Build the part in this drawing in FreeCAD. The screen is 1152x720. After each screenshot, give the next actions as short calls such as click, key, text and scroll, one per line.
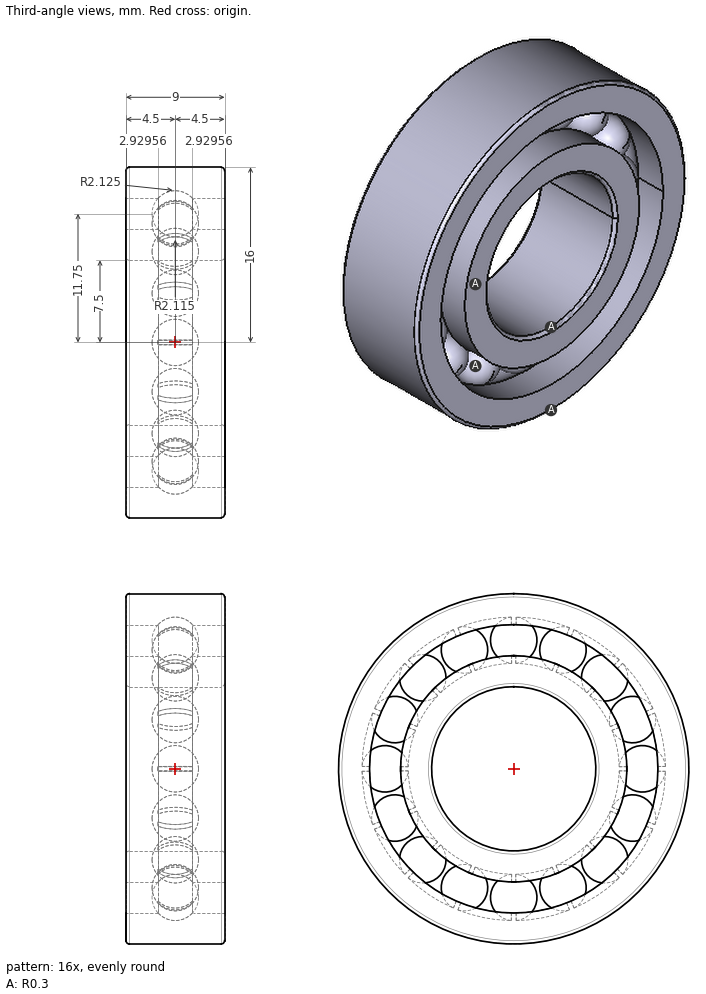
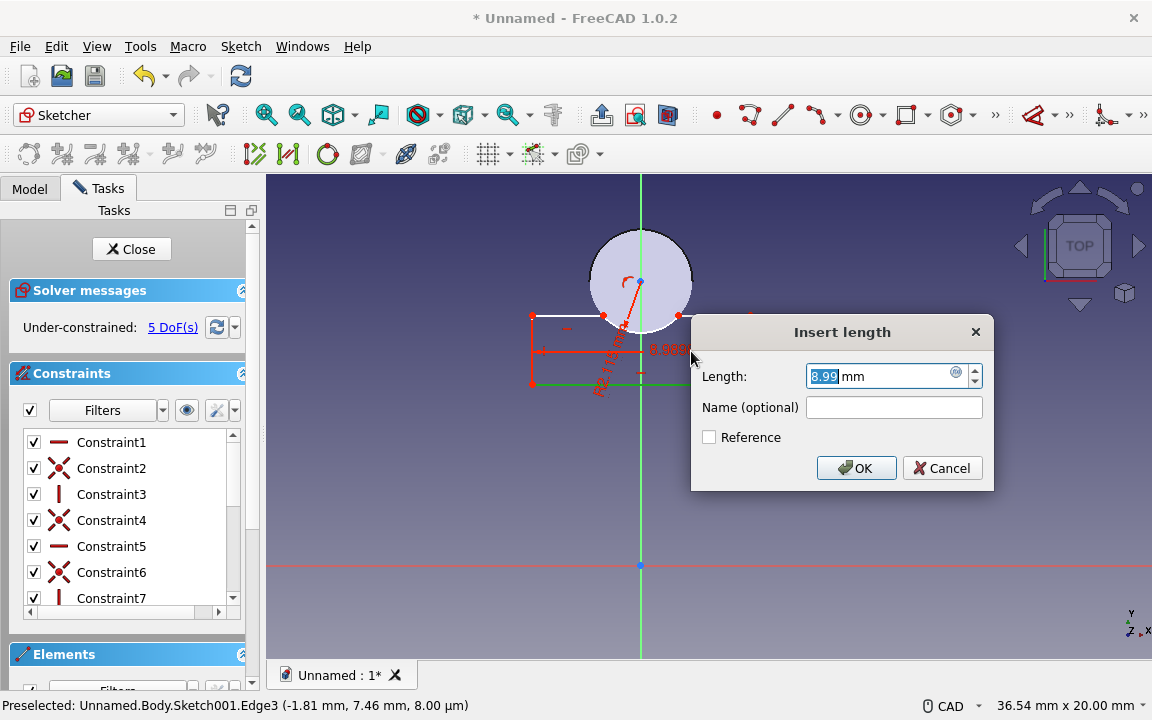
text(9)
key(Return)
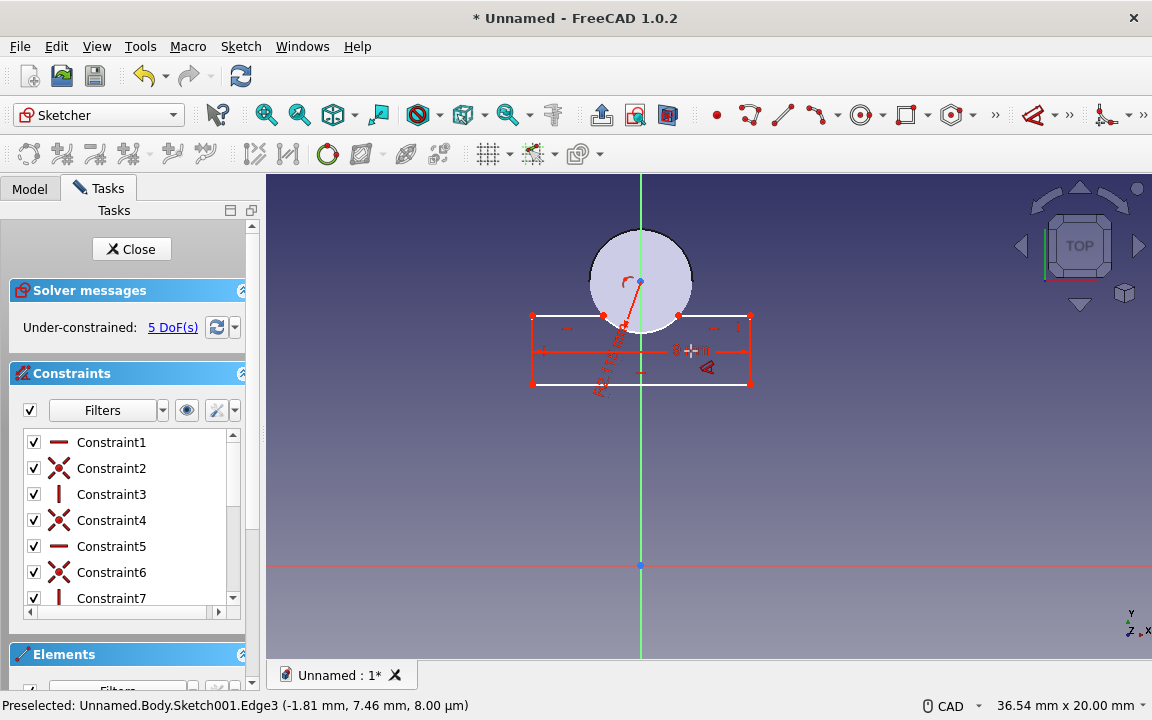
click(532, 316)
click(586, 600)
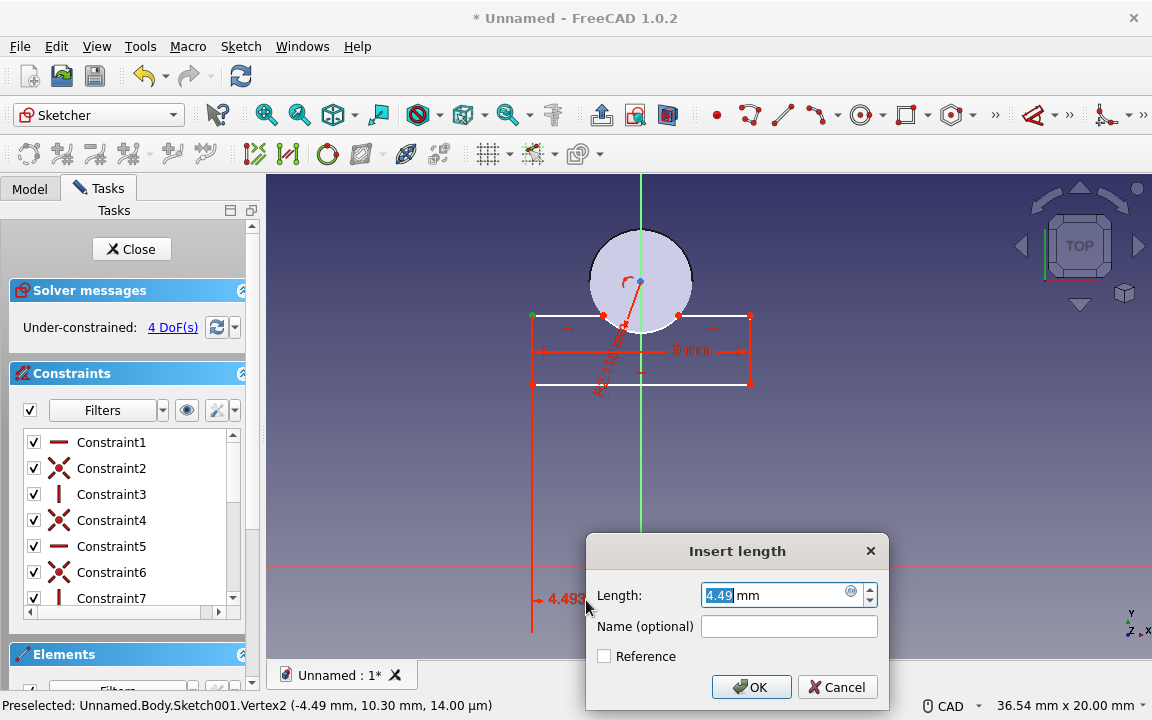
text(4.5)
key(Return)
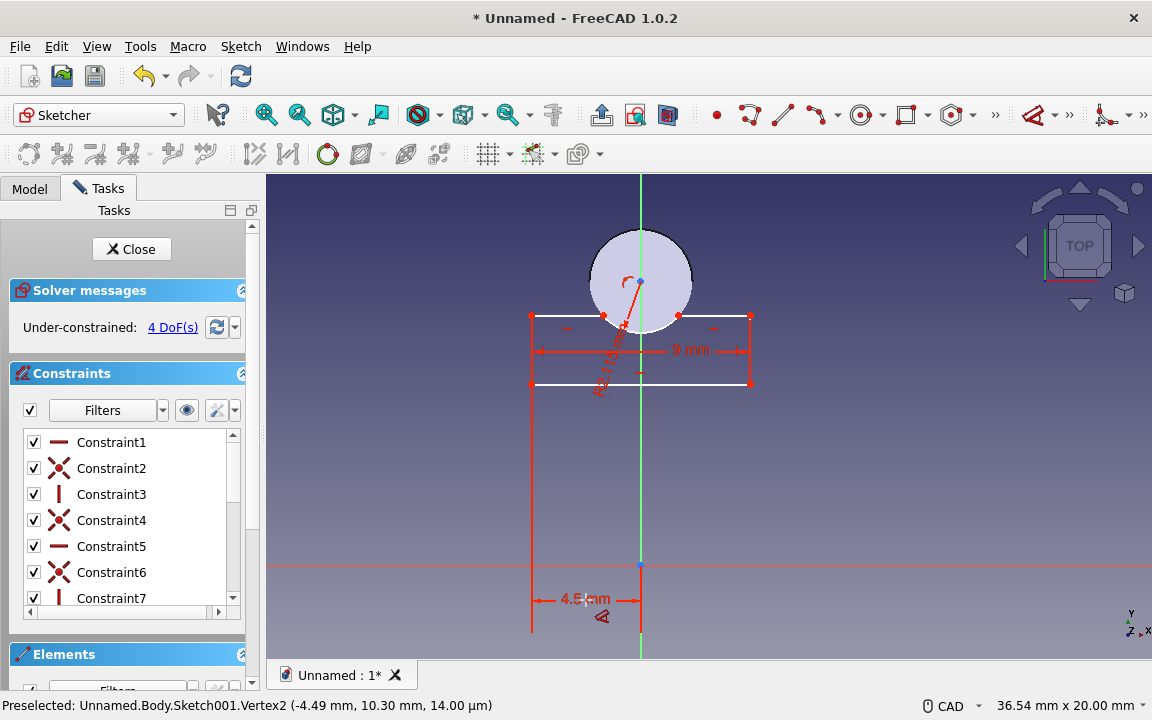
click(532, 385)
click(498, 475)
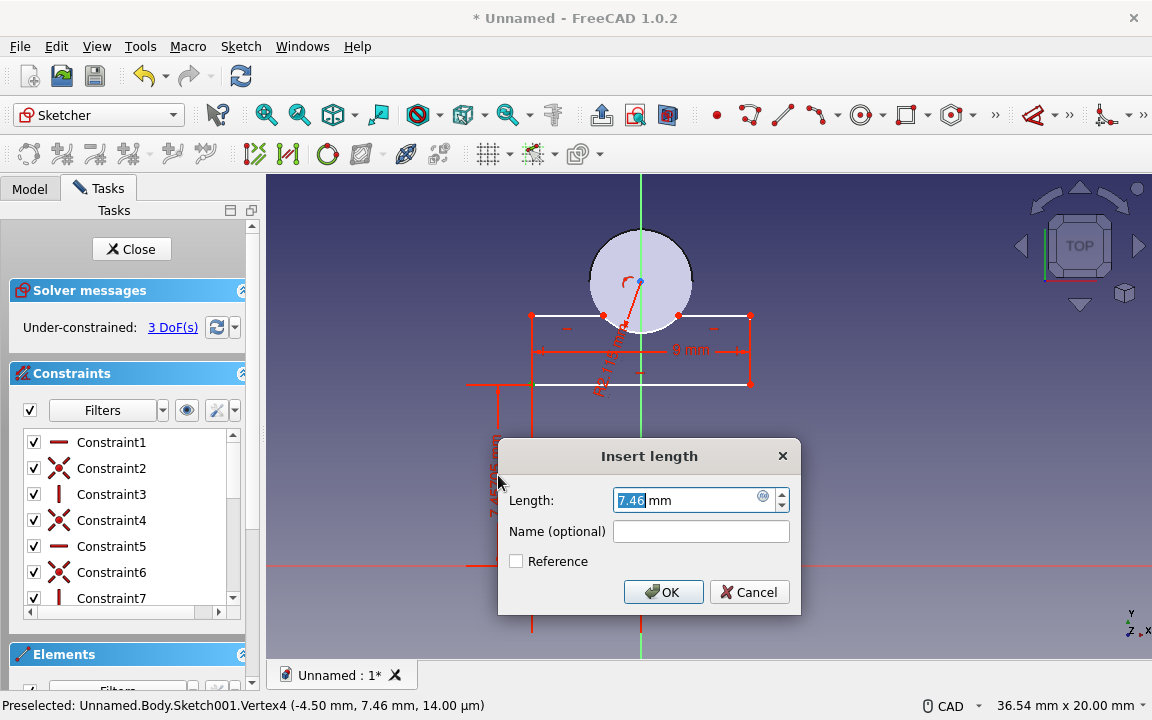
text(7.5)
key(Return)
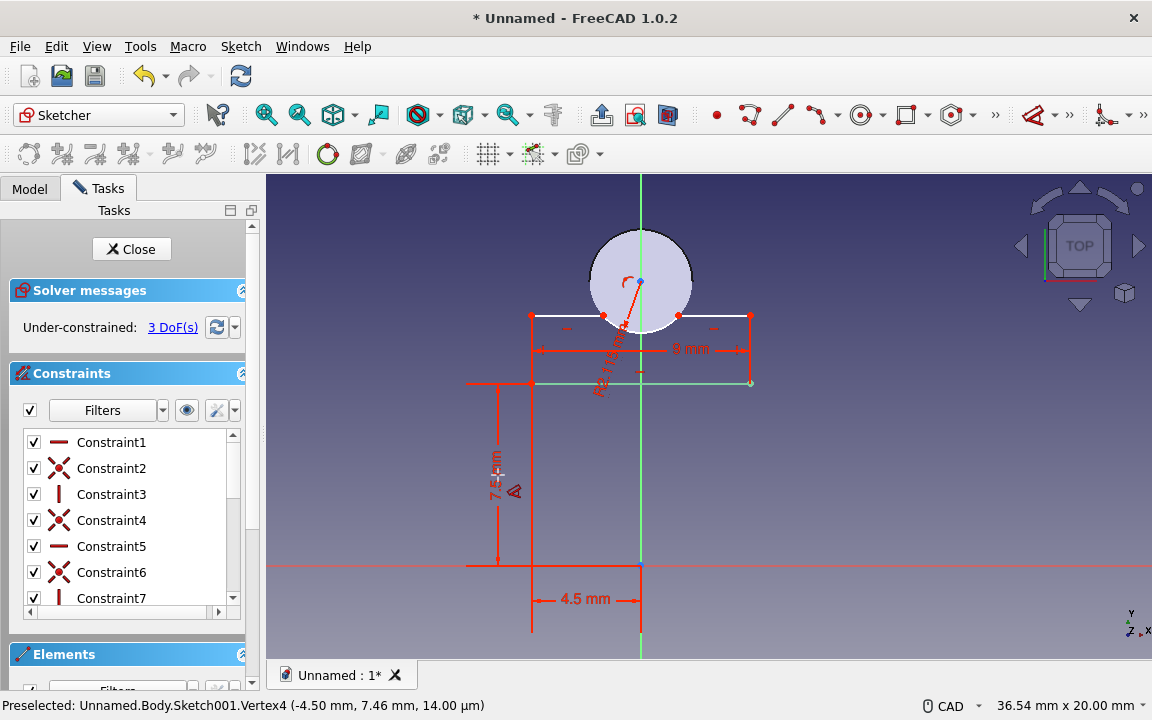
click(641, 282)
click(675, 424)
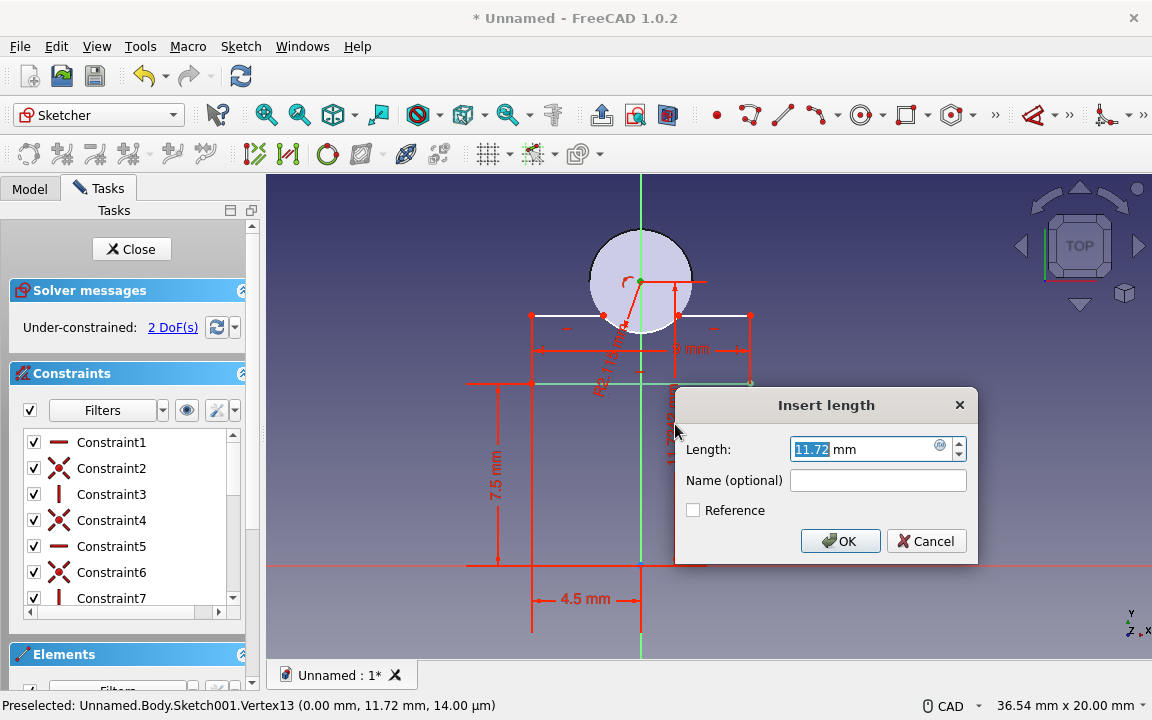
text(11.75)
key(Return)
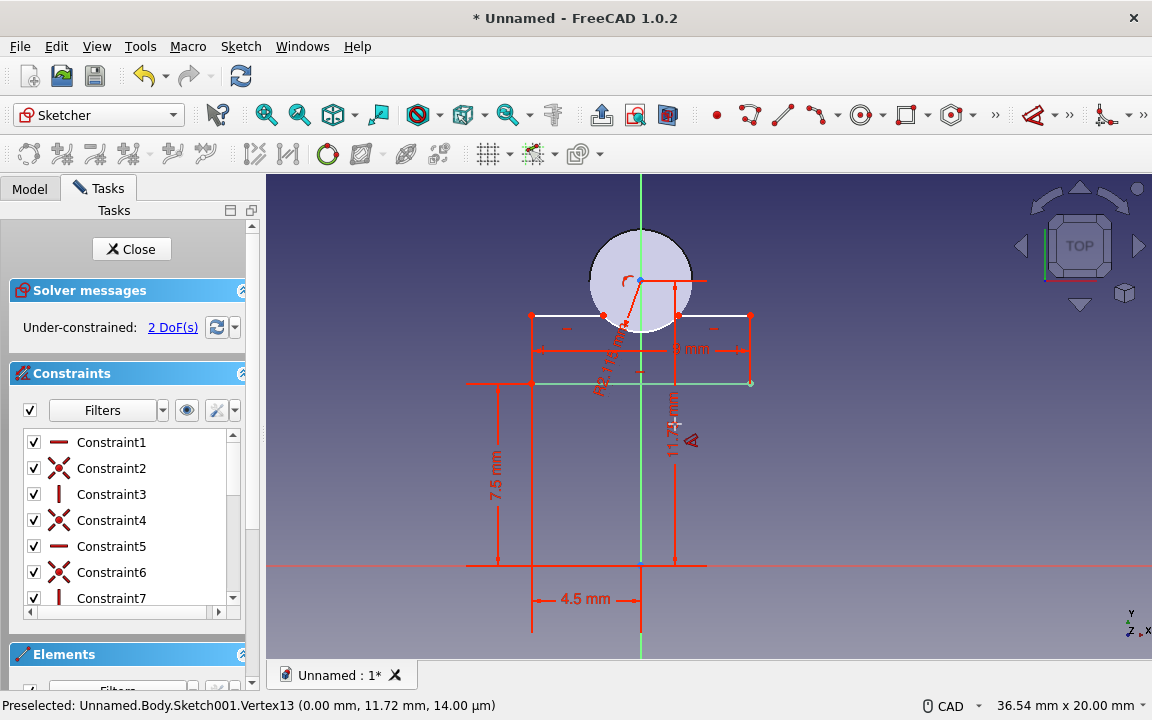
click(582, 316)
click(568, 282)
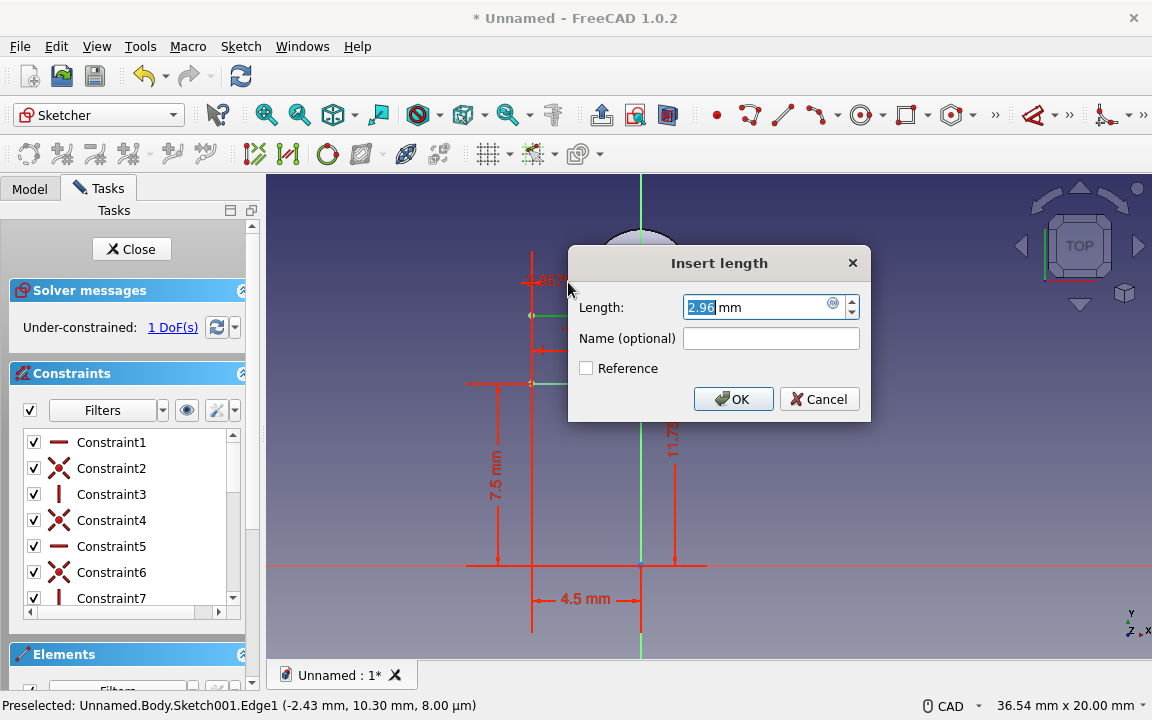
text(2.92956)
key(Return)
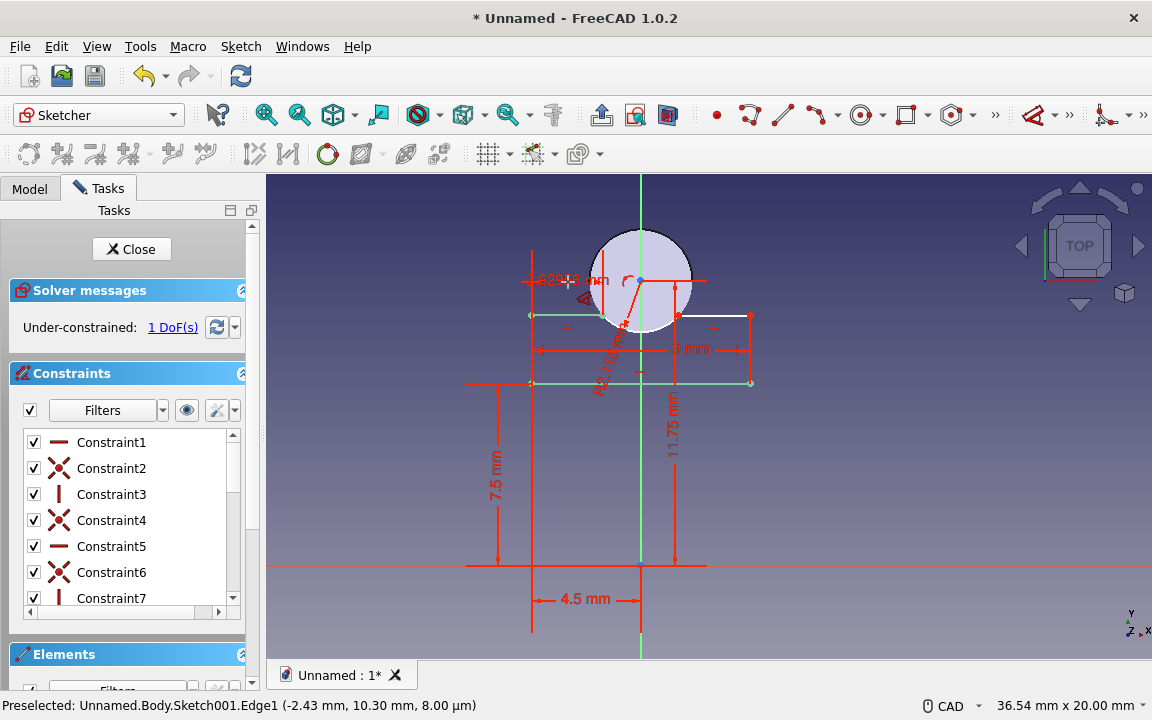
click(729, 316)
click(714, 282)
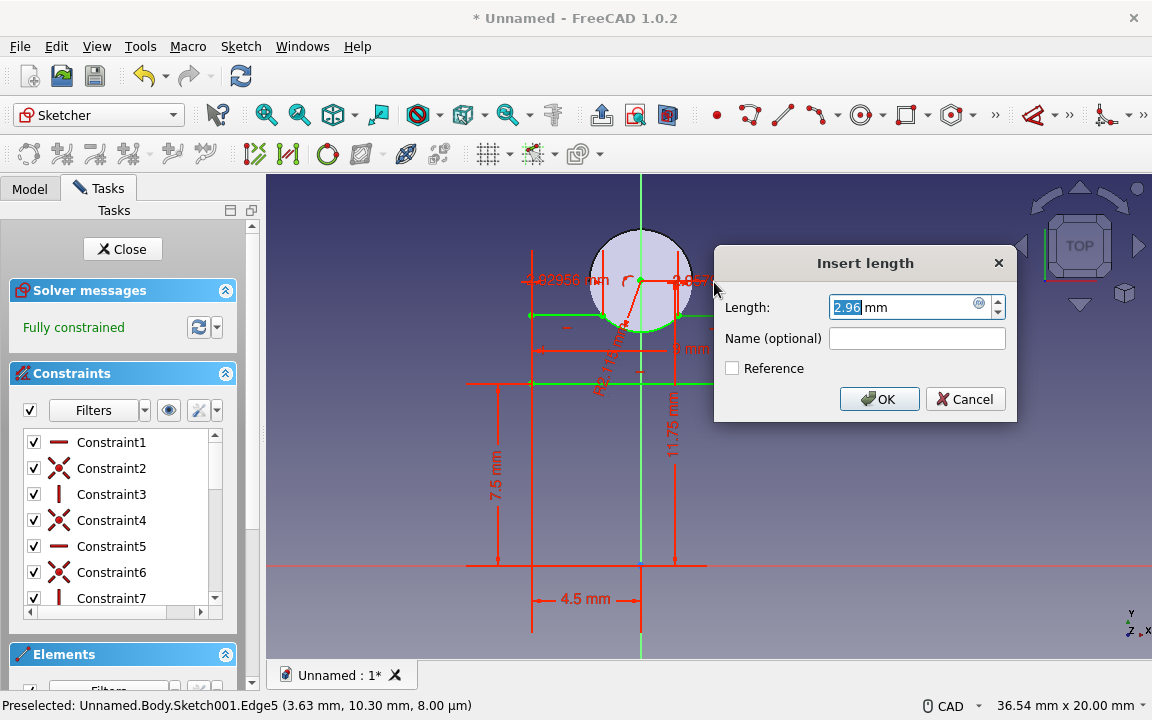
text(2.92956)
key(Return)
key(Escape)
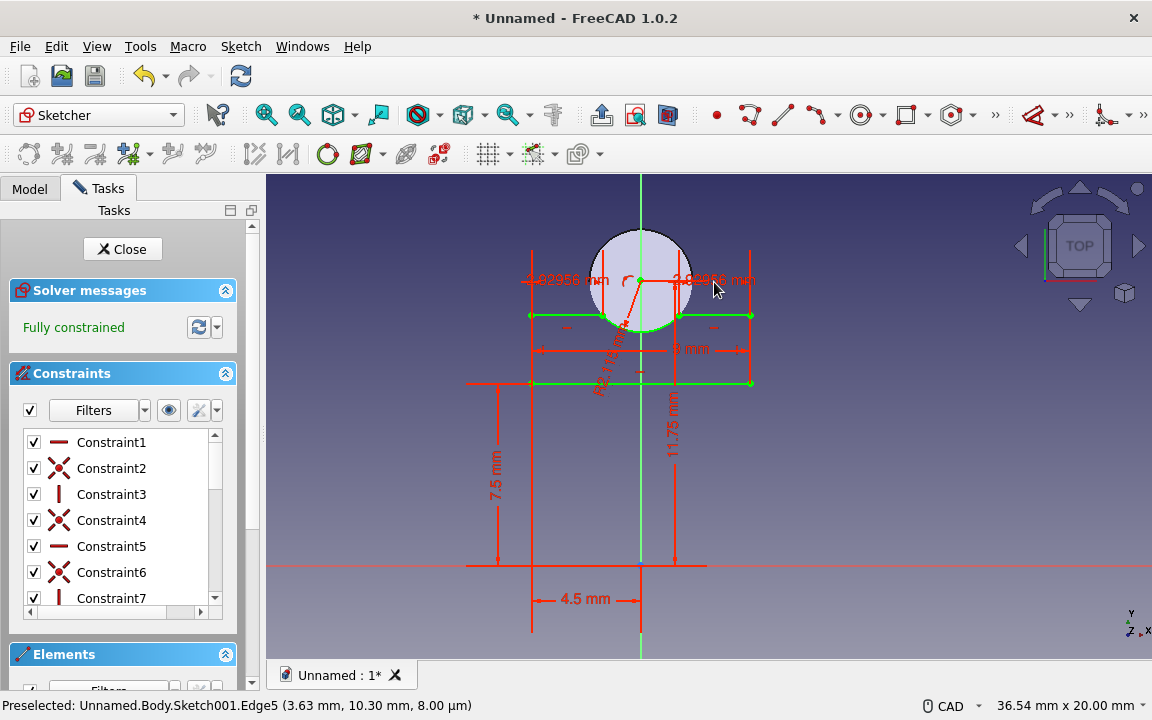
click(123, 249)